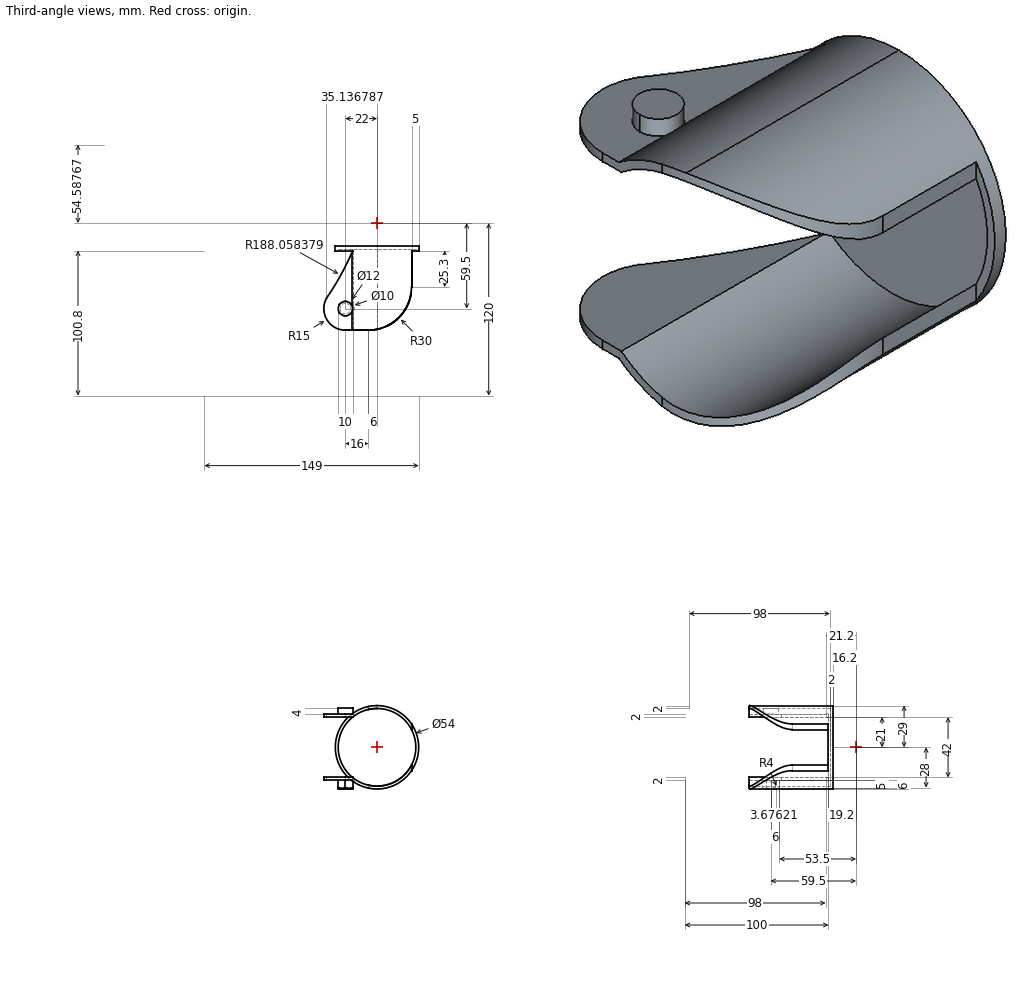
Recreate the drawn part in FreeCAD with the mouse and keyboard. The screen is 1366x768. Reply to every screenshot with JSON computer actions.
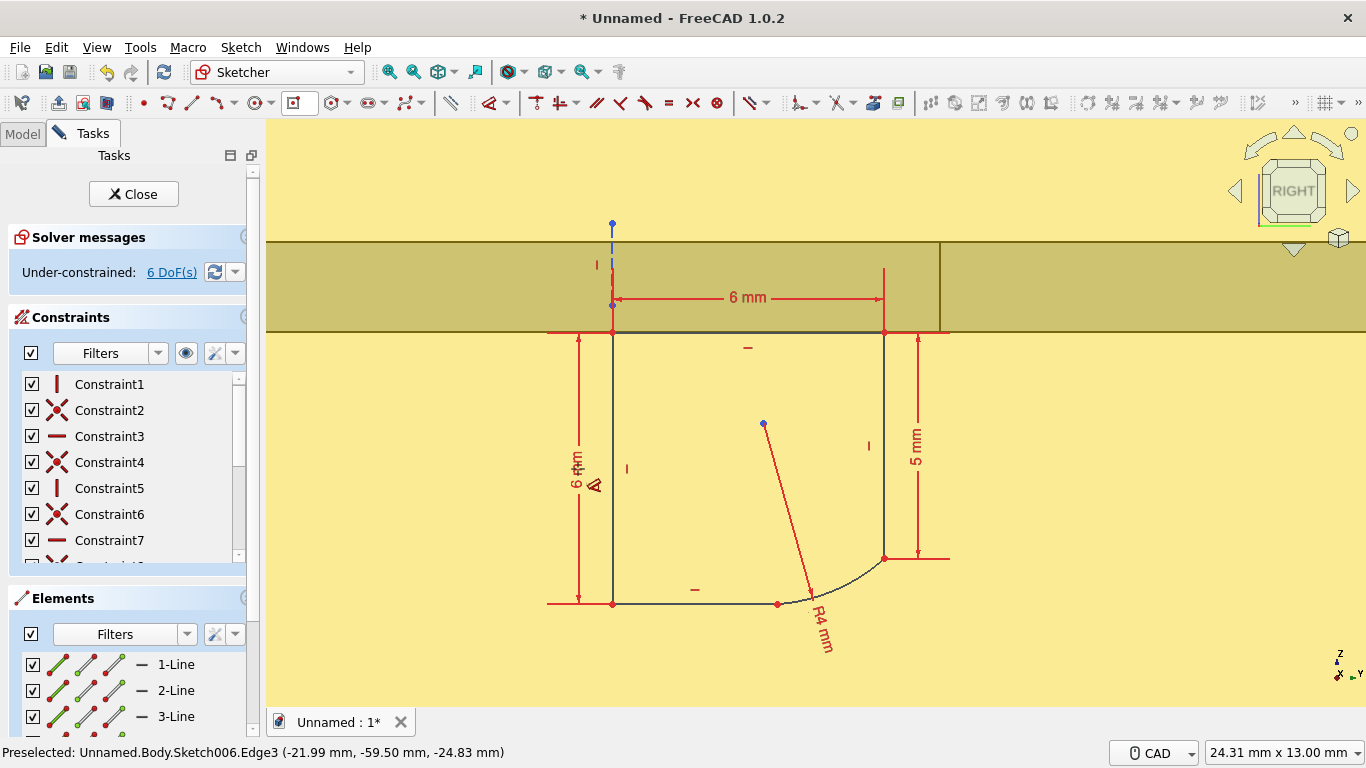
{"action": "left_click", "coordinate": [884, 559]}
{"action": "left_click", "coordinate": [850, 353]}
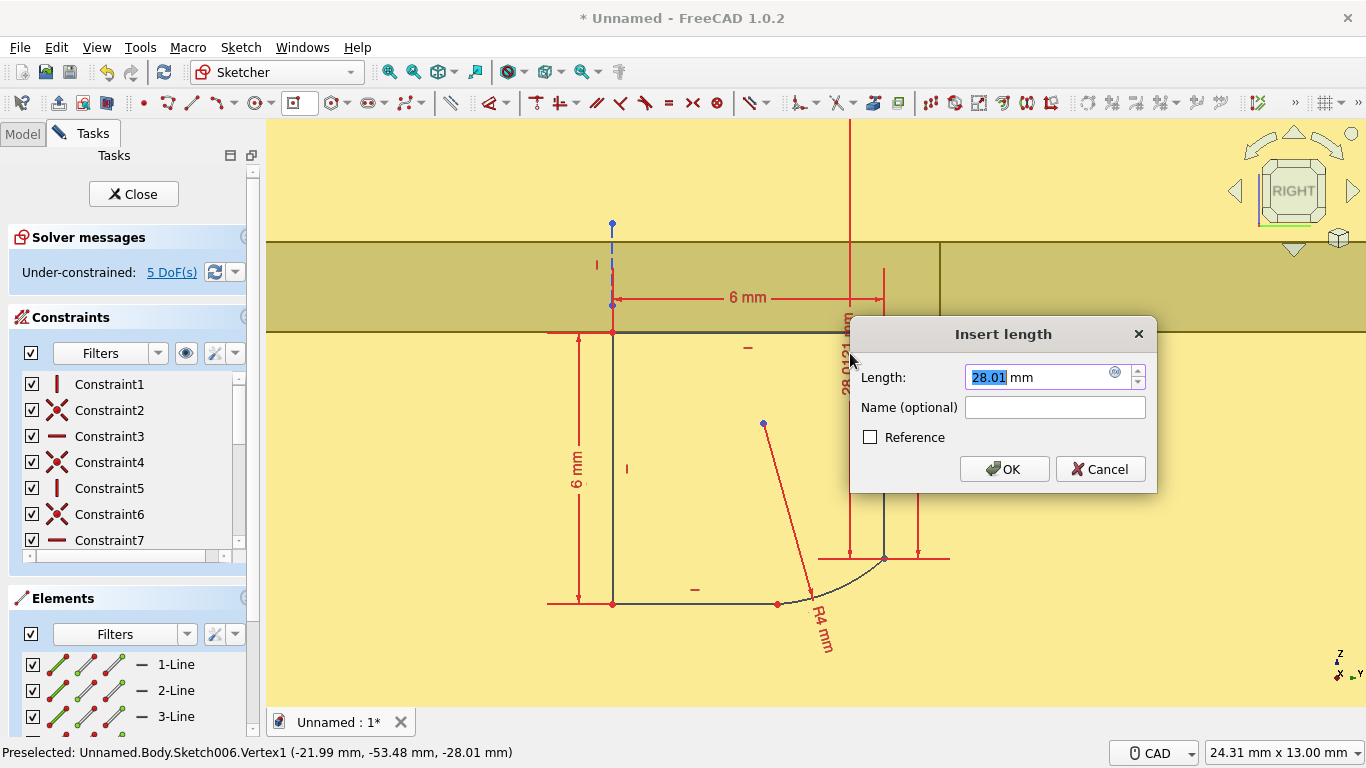
{"action": "type", "text": "28"}
{"action": "key", "text": "Return"}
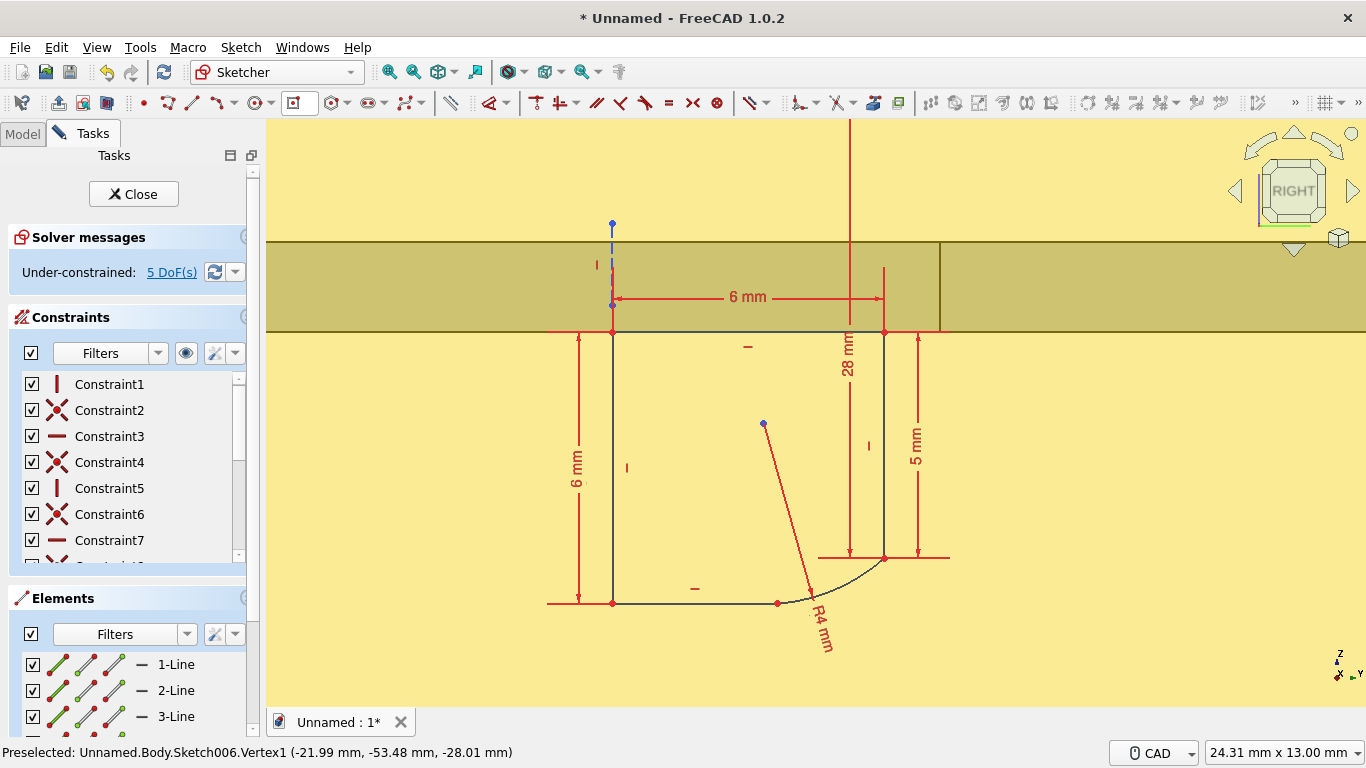
{"action": "left_click", "coordinate": [884, 558]}
{"action": "left_click", "coordinate": [1043, 592]}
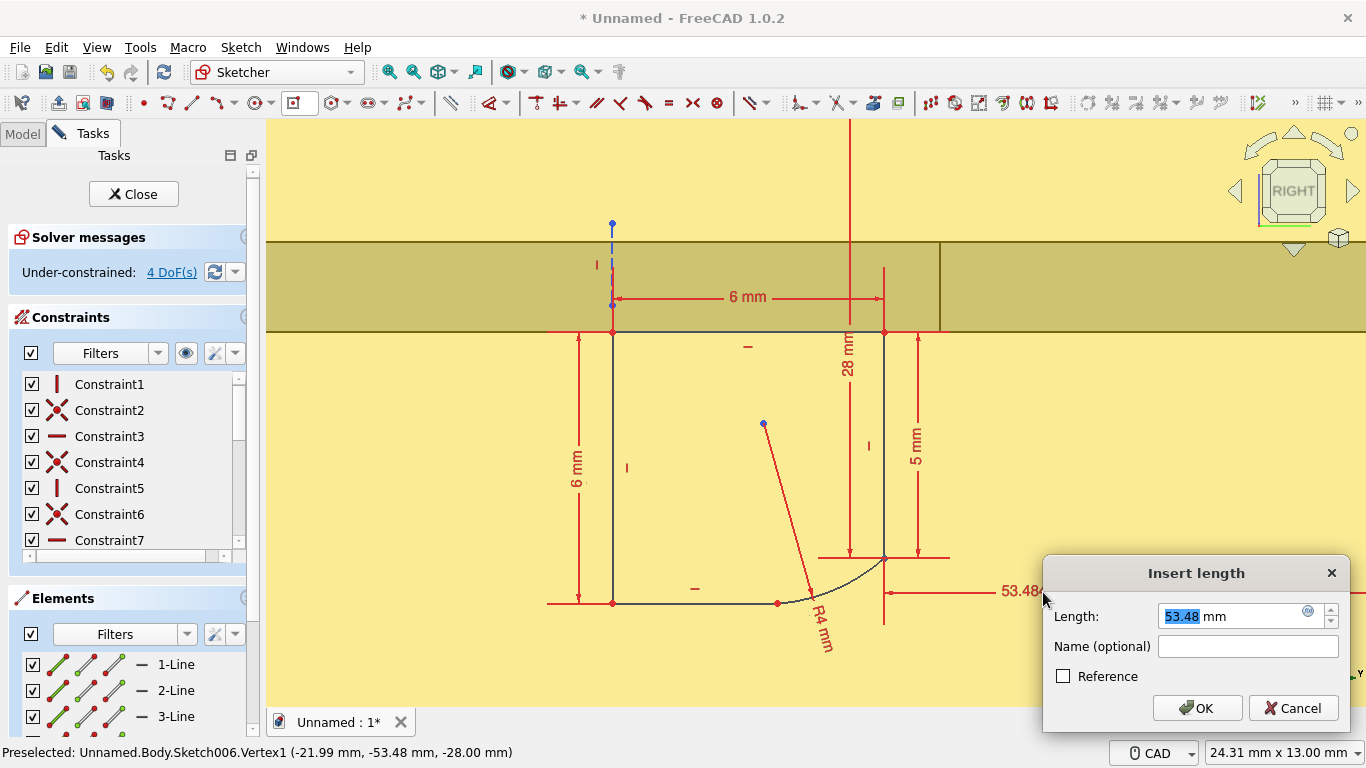
{"action": "type", "text": "53.5"}
{"action": "key", "text": "Return"}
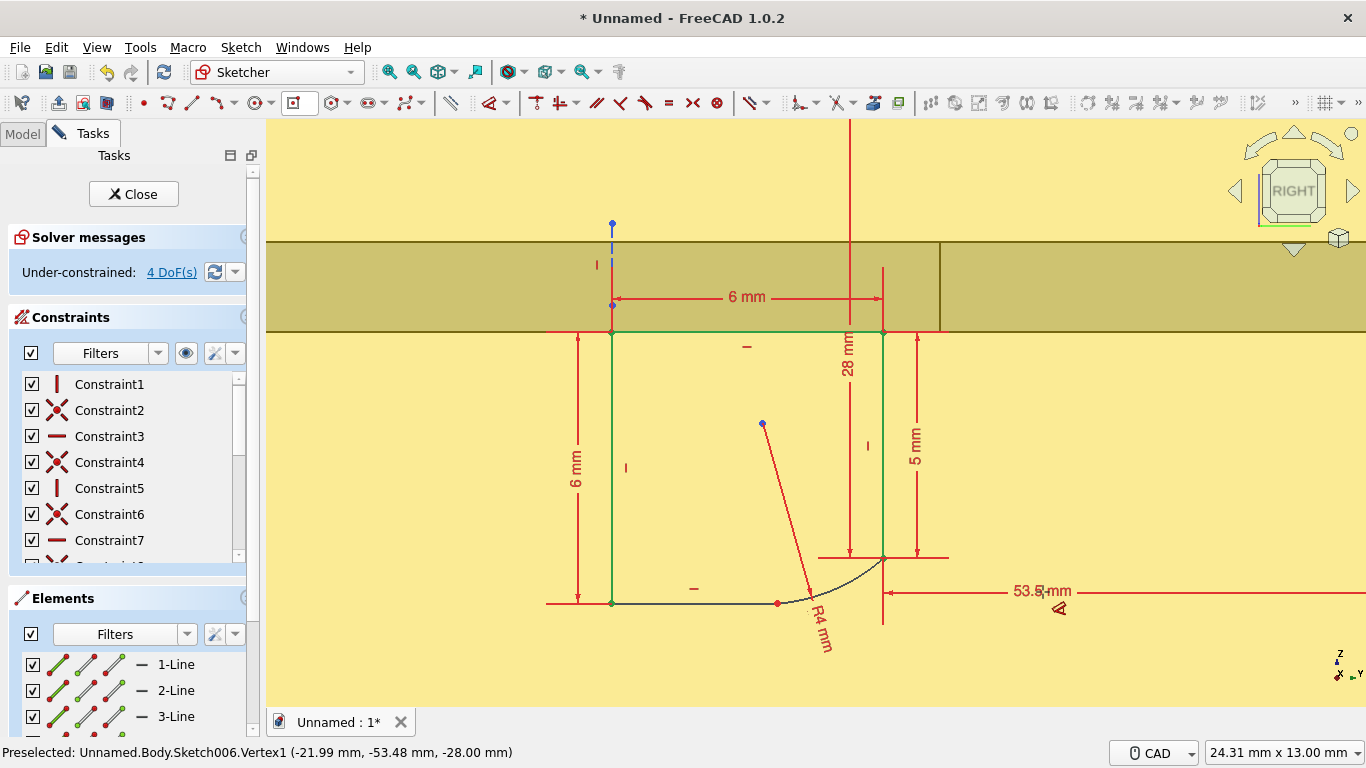
{"action": "left_click", "coordinate": [612, 306]}
{"action": "left_click", "coordinate": [1042, 340]}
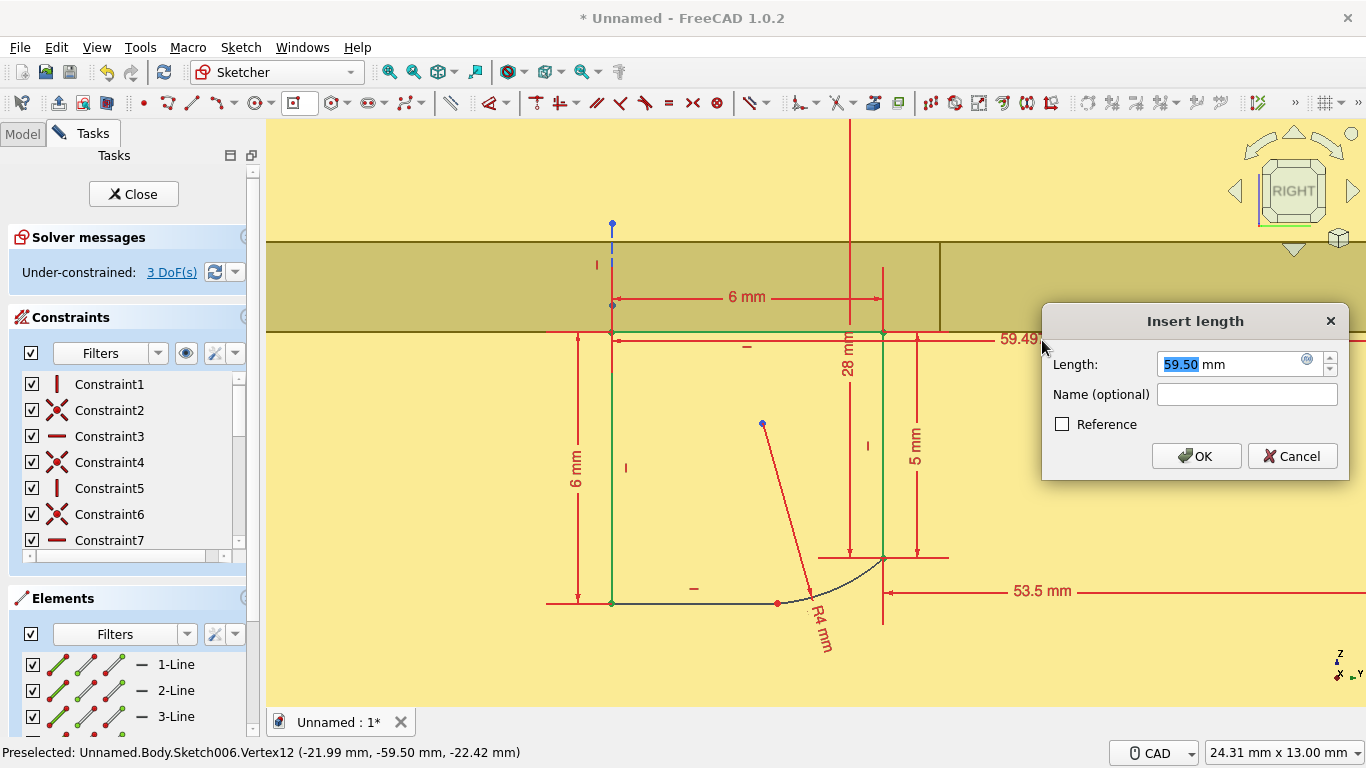
{"action": "type", "text": "59.5"}
{"action": "key", "text": "Return"}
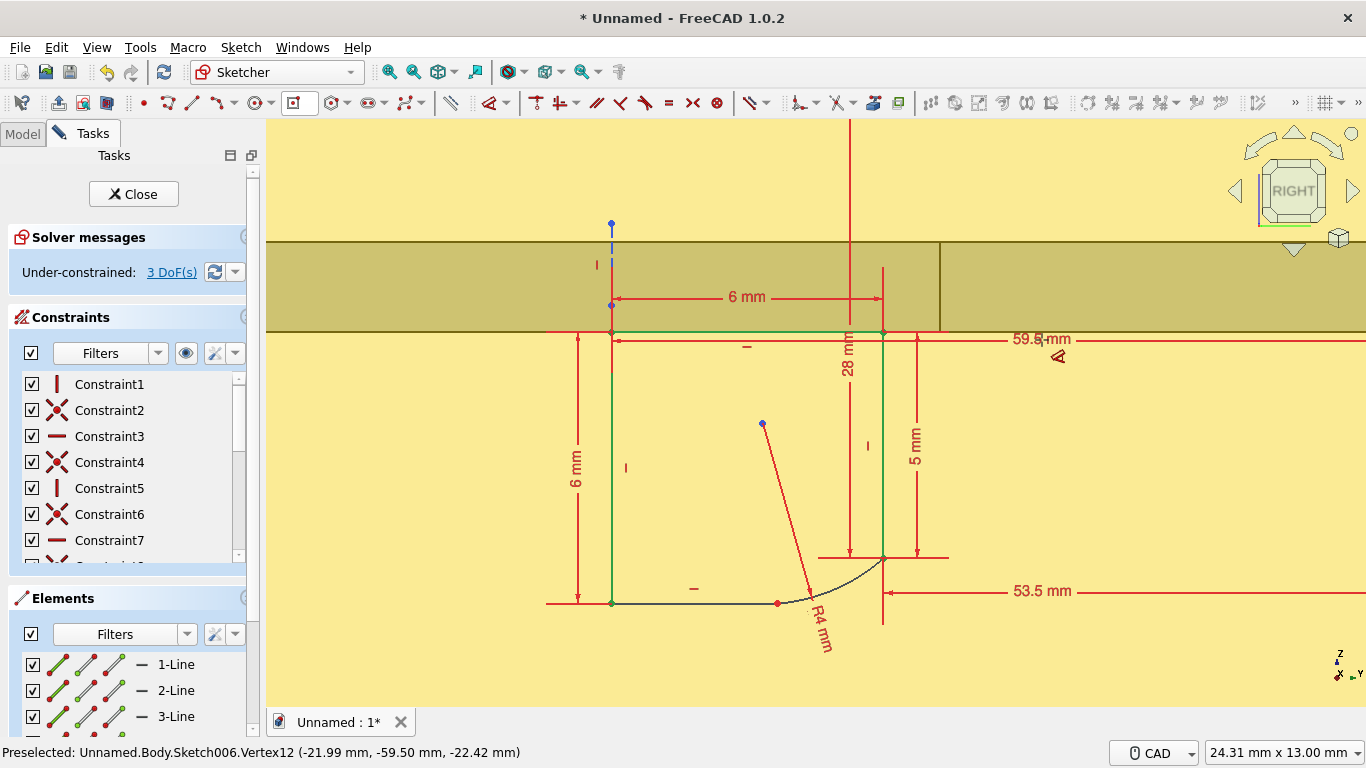
{"action": "left_click", "coordinate": [662, 604]}
{"action": "left_click", "coordinate": [695, 638]}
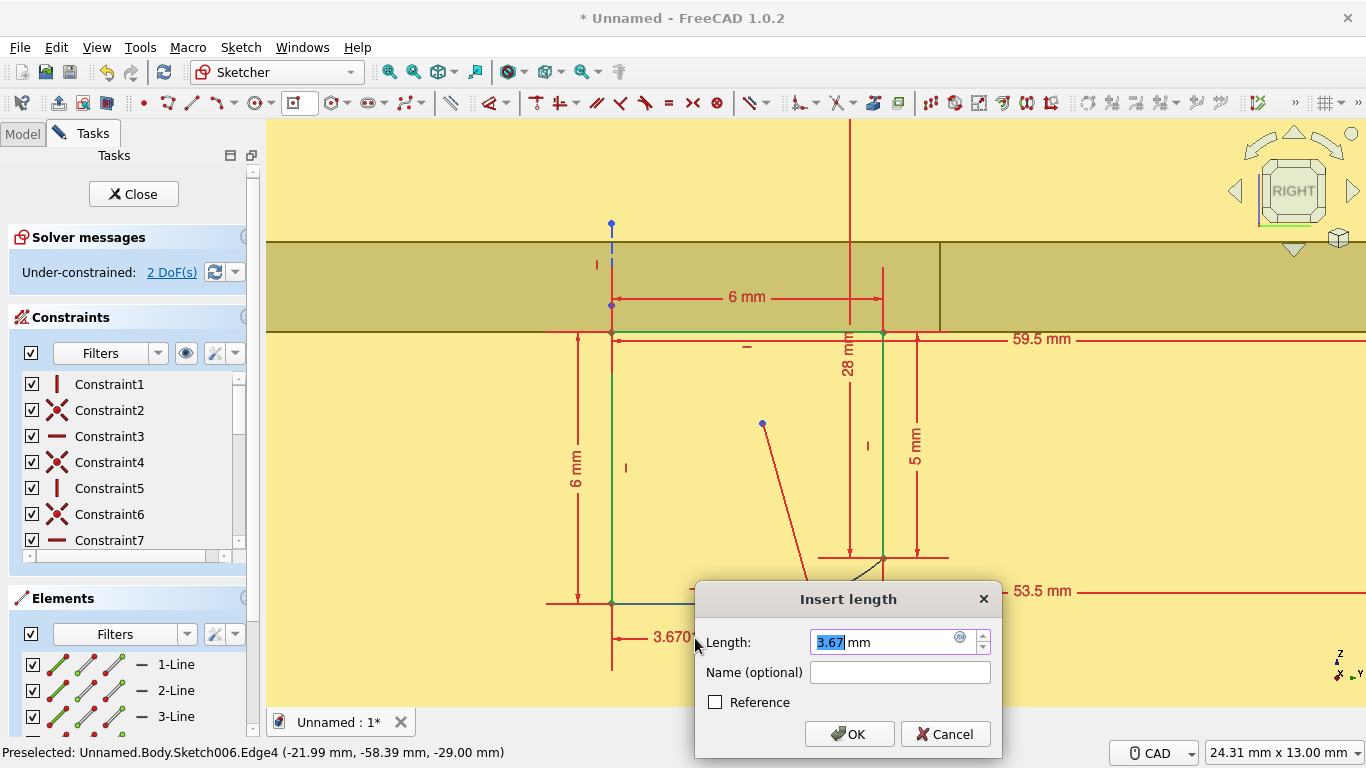
{"action": "type", "text": "3.67621"}
{"action": "key", "text": "Return"}
{"action": "key", "text": "Escape"}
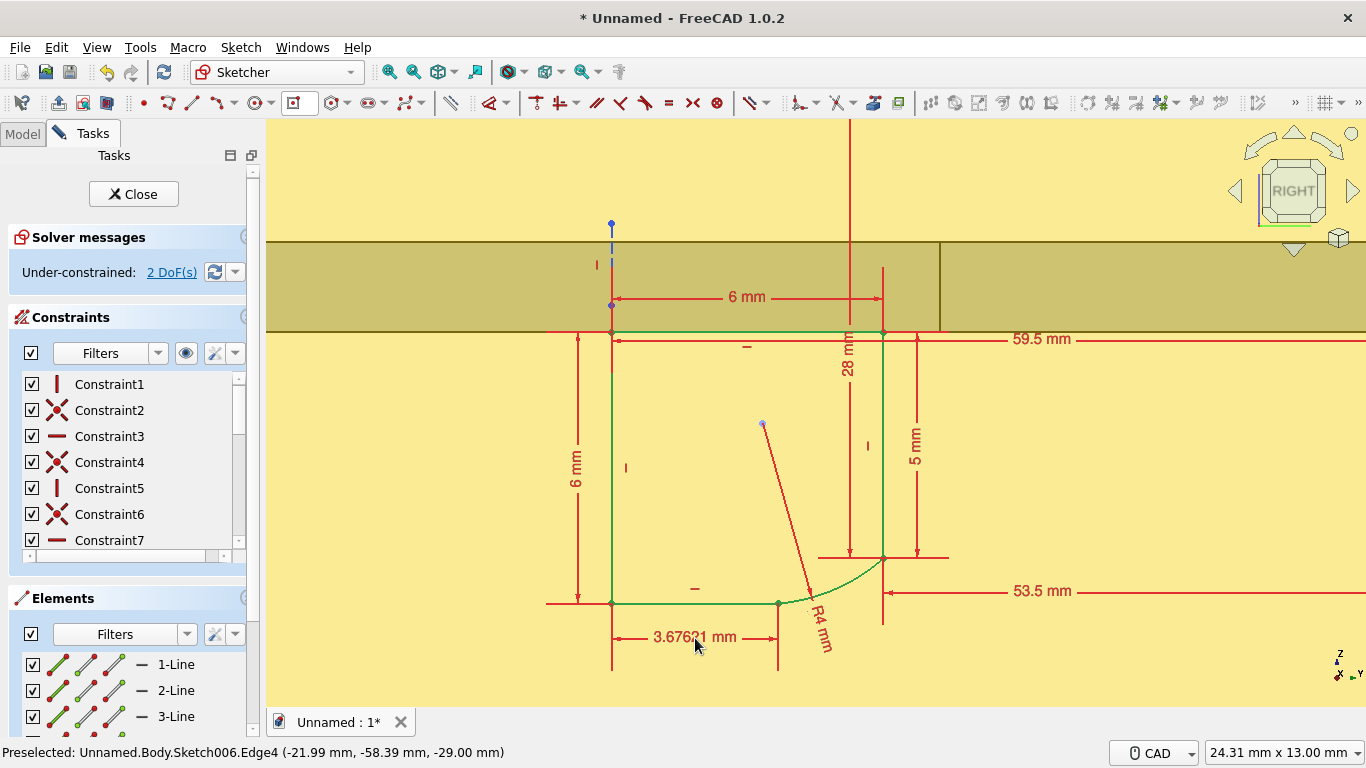
{"action": "left_click", "coordinate": [134, 194]}